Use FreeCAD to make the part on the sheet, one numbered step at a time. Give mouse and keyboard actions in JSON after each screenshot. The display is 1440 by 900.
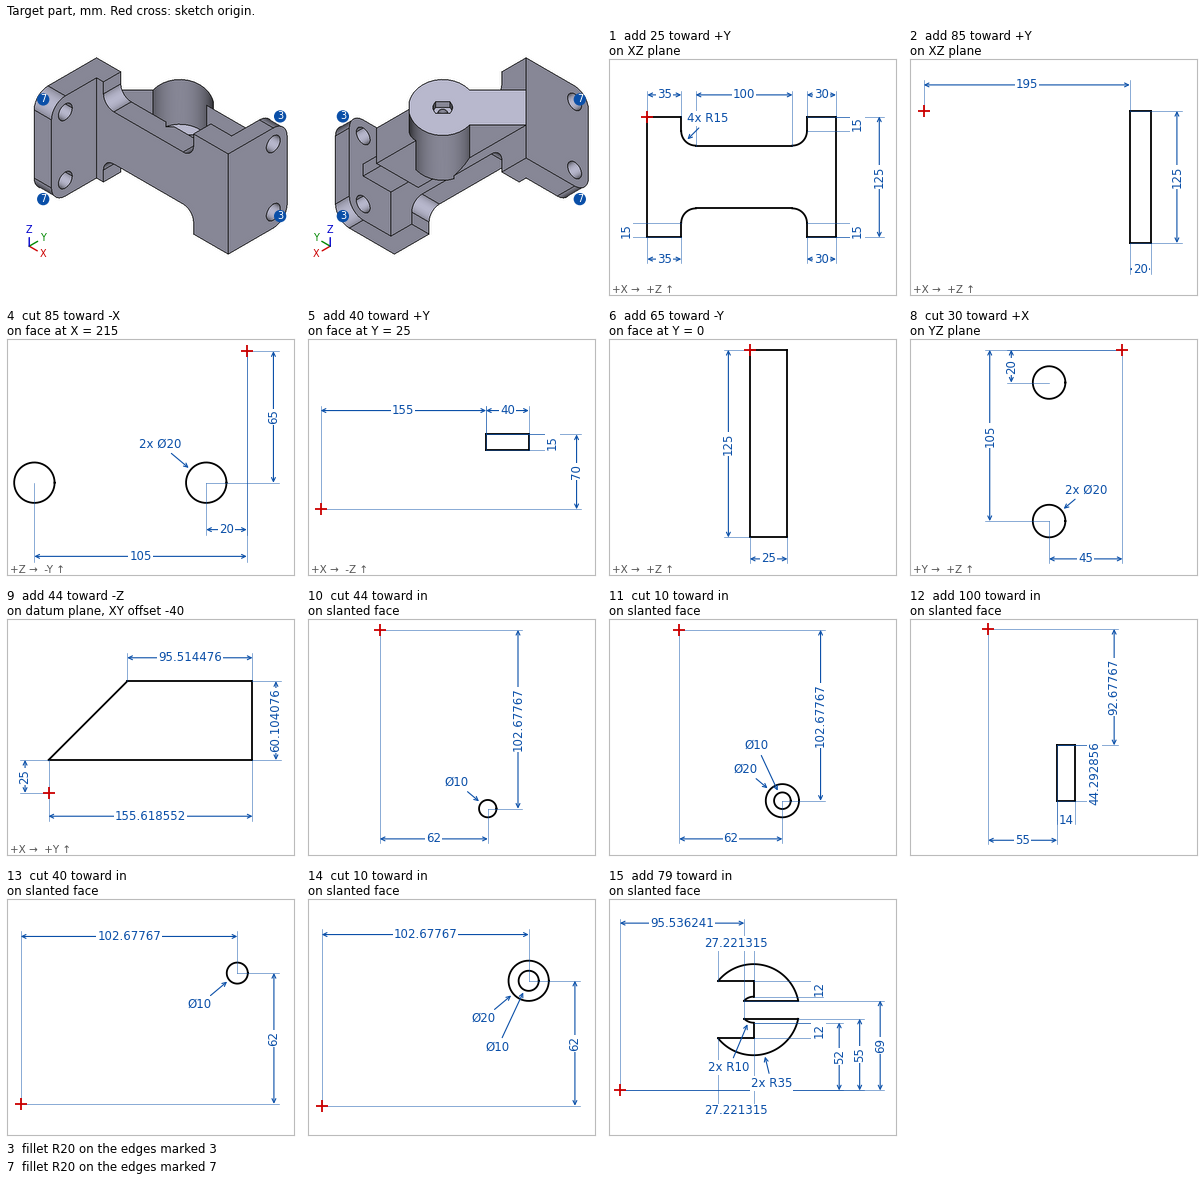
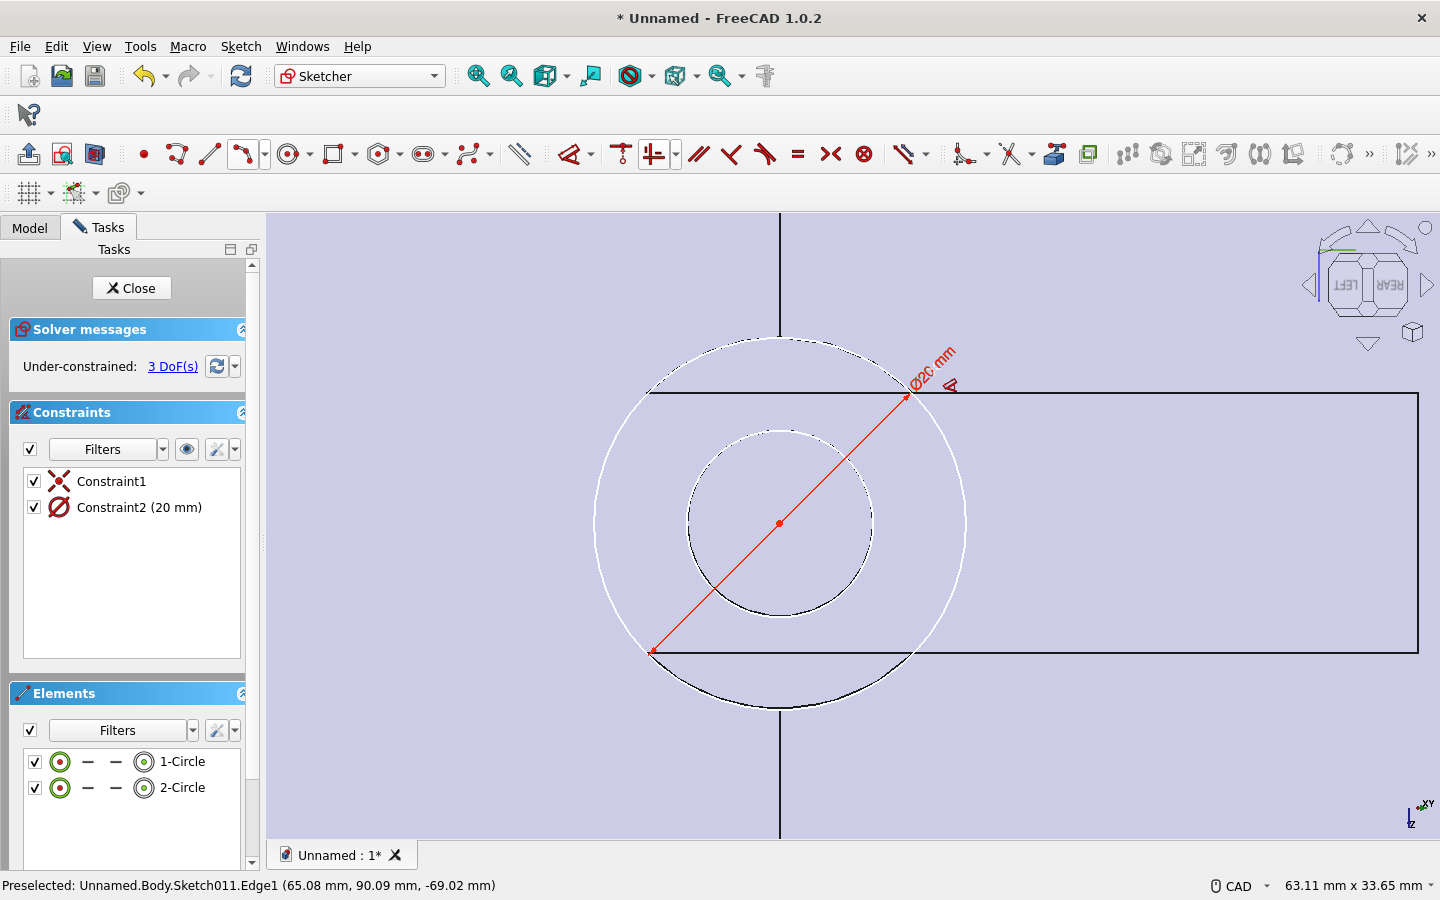
{"action": "left_click", "coordinate": [846, 458]}
{"action": "left_click", "coordinate": [869, 435]}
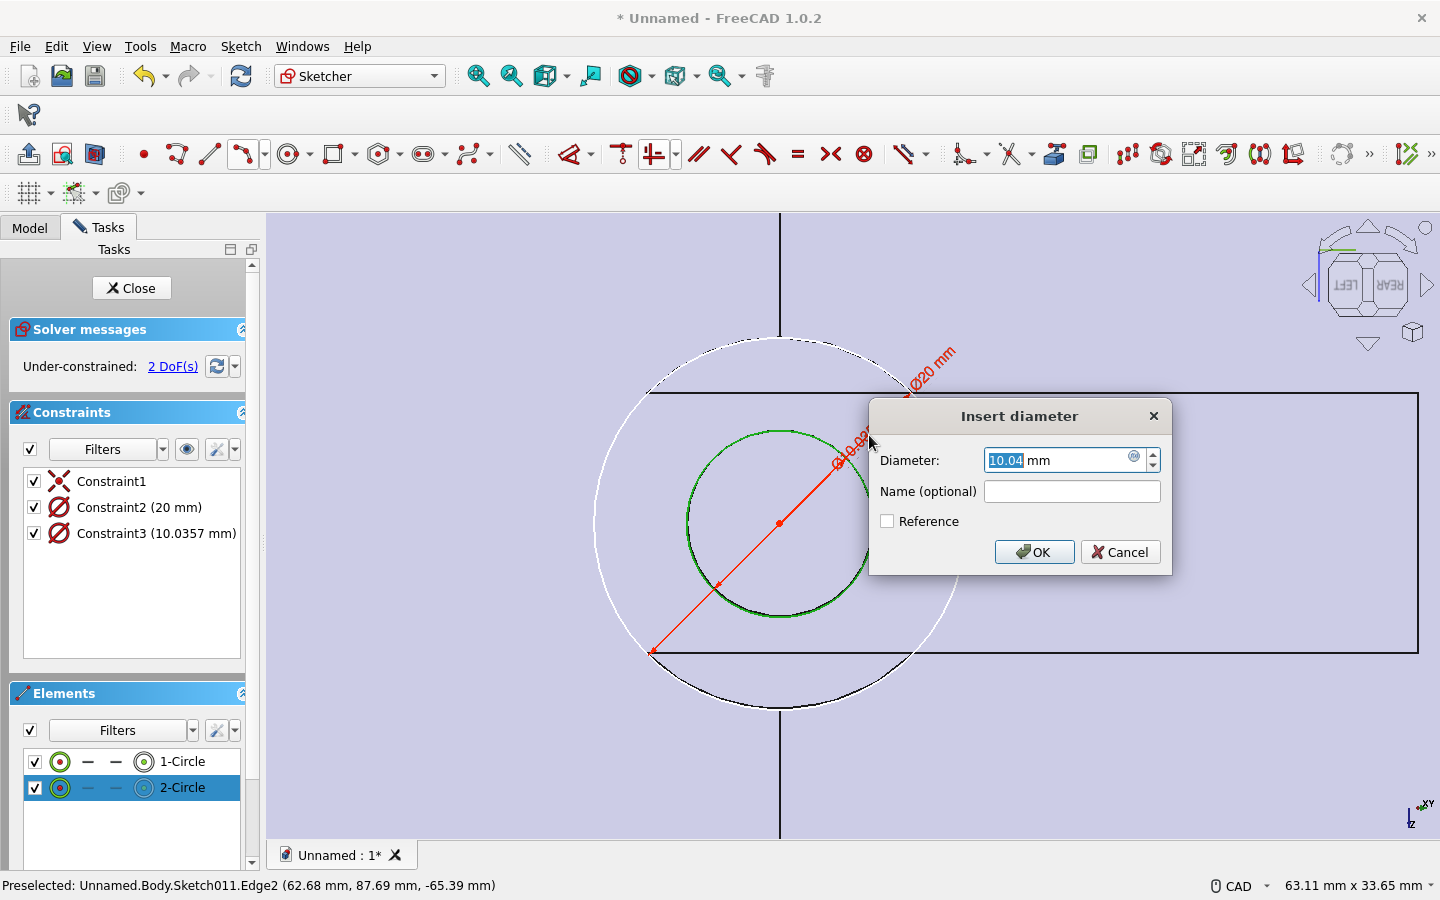
{"action": "type", "text": "10"}
{"action": "key", "text": "Return"}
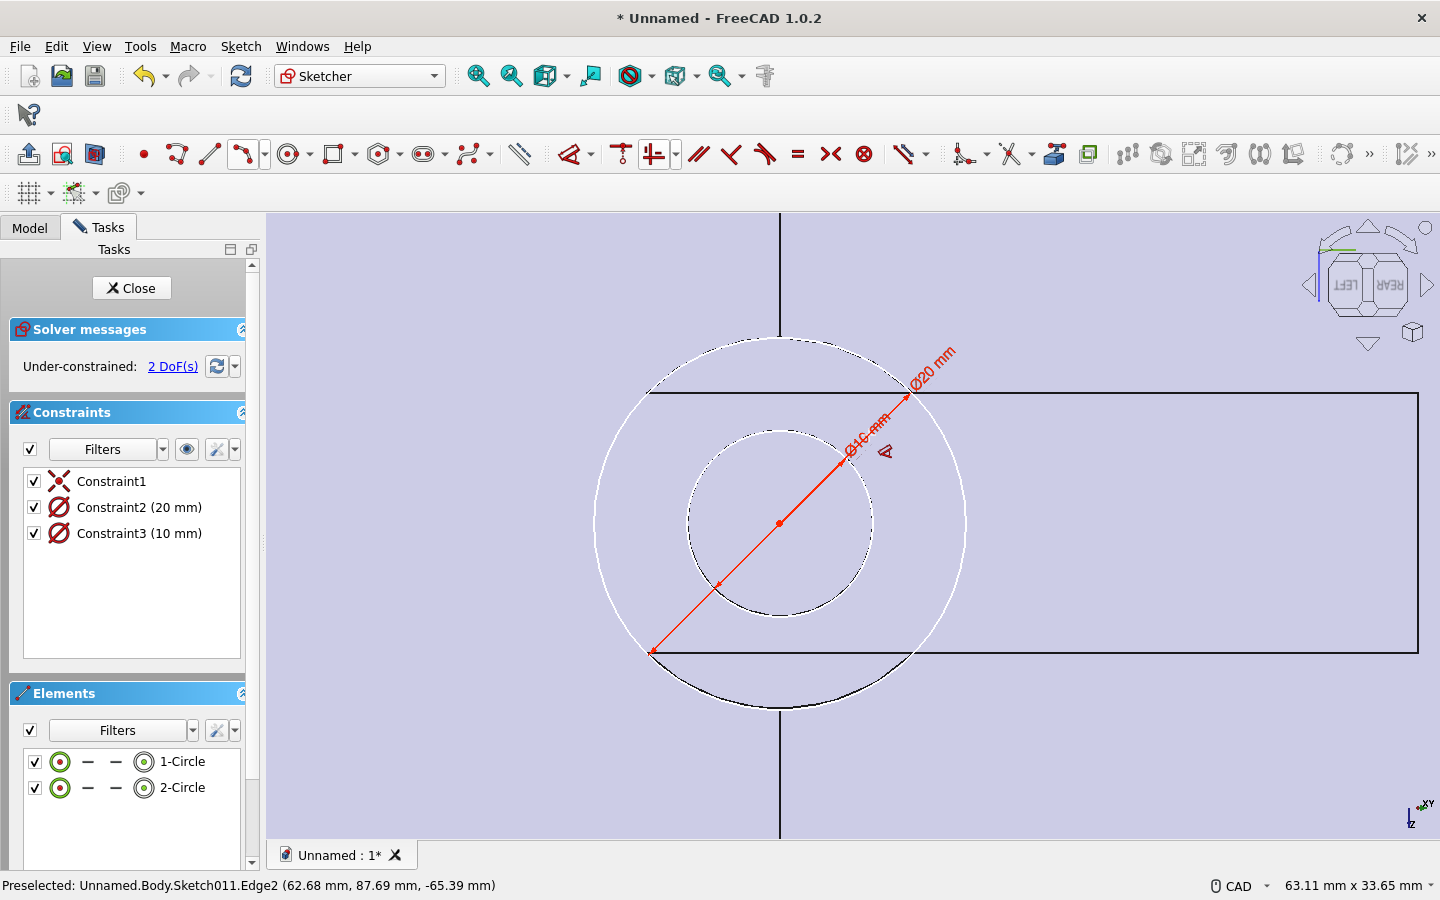
{"action": "left_click", "coordinate": [780, 524]}
{"action": "left_click", "coordinate": [814, 667]}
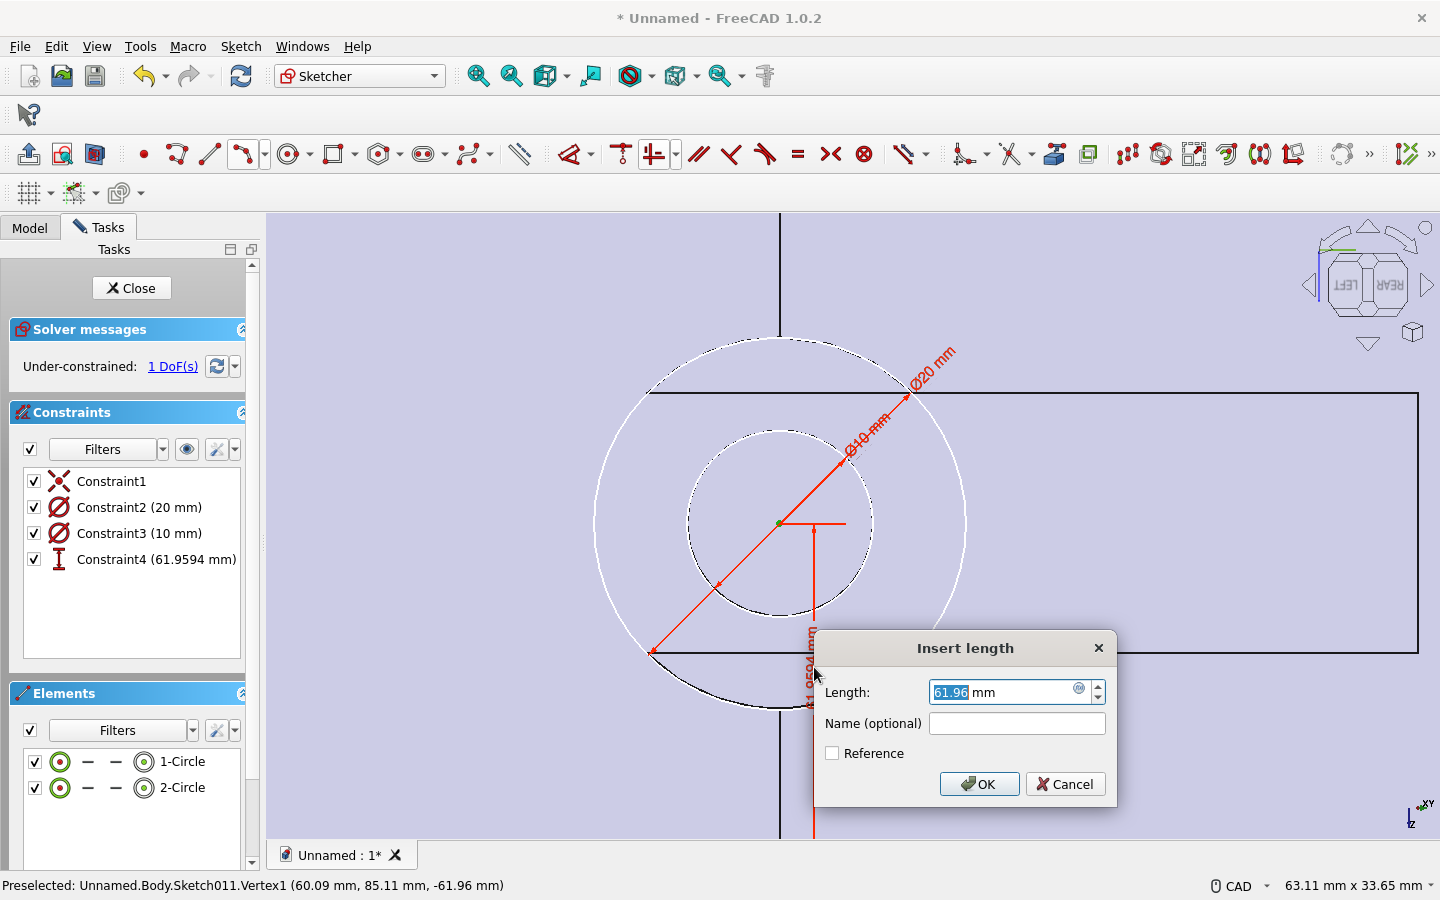
{"action": "type", "text": "62"}
{"action": "key", "text": "Return"}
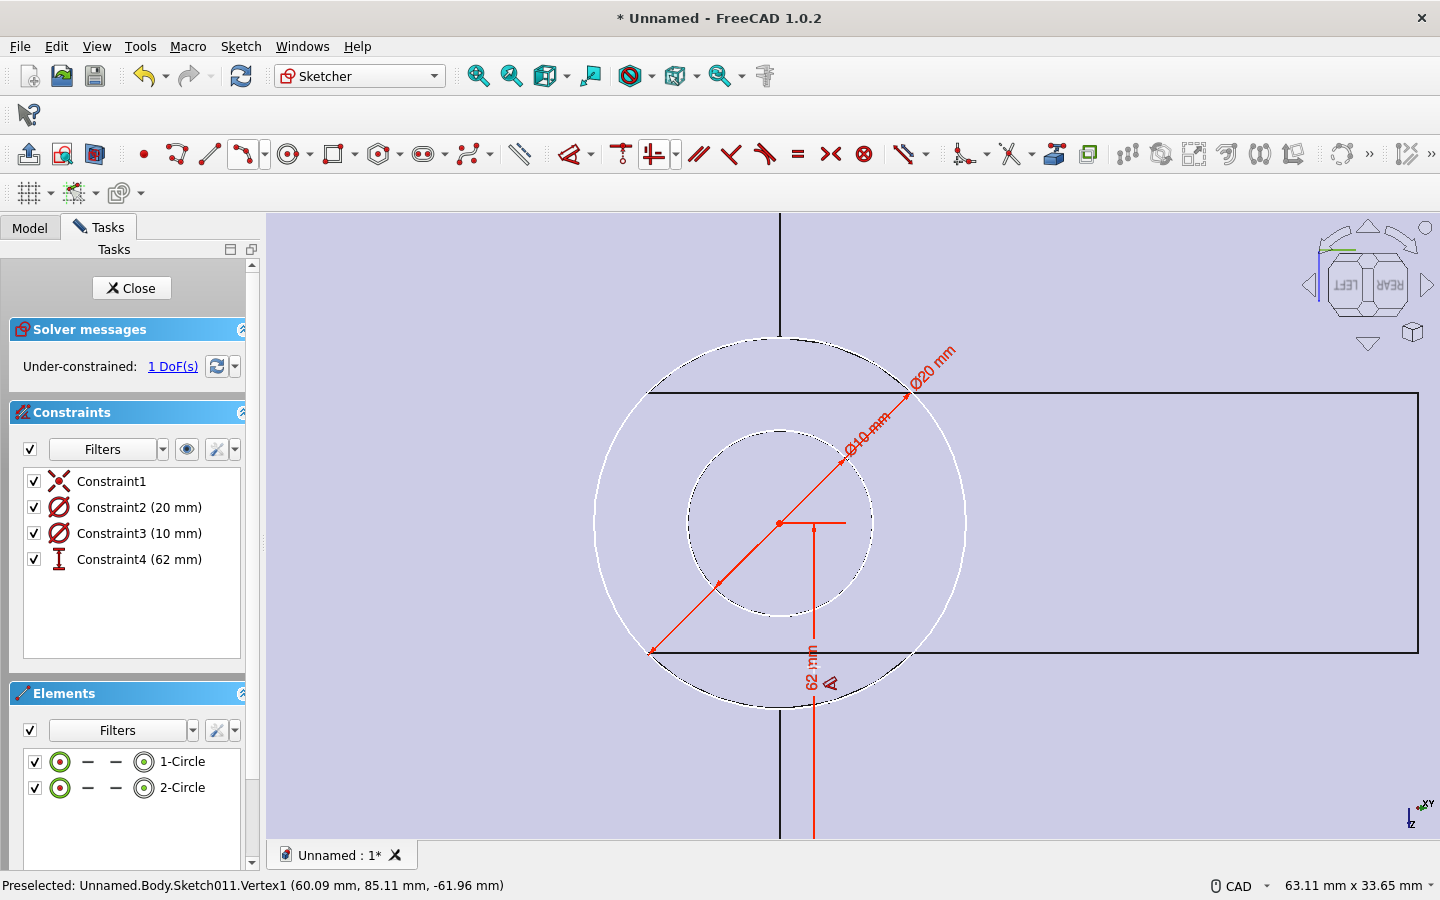
{"action": "left_click", "coordinate": [780, 523]}
{"action": "left_click", "coordinate": [537, 489]}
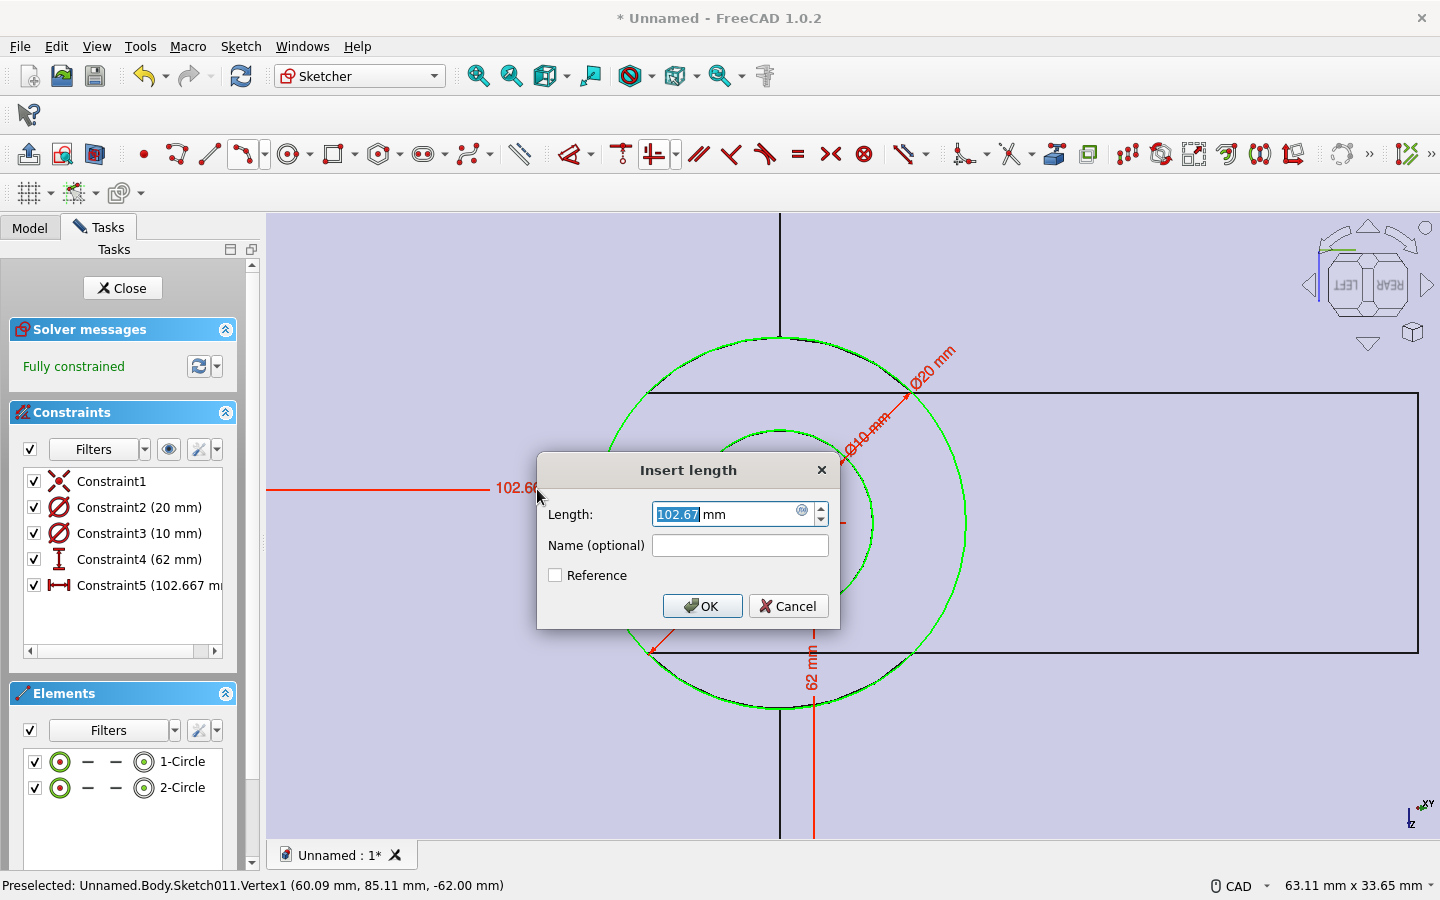
{"action": "type", "text": "102.67767"}
{"action": "key", "text": "Return"}
{"action": "key", "text": "Escape"}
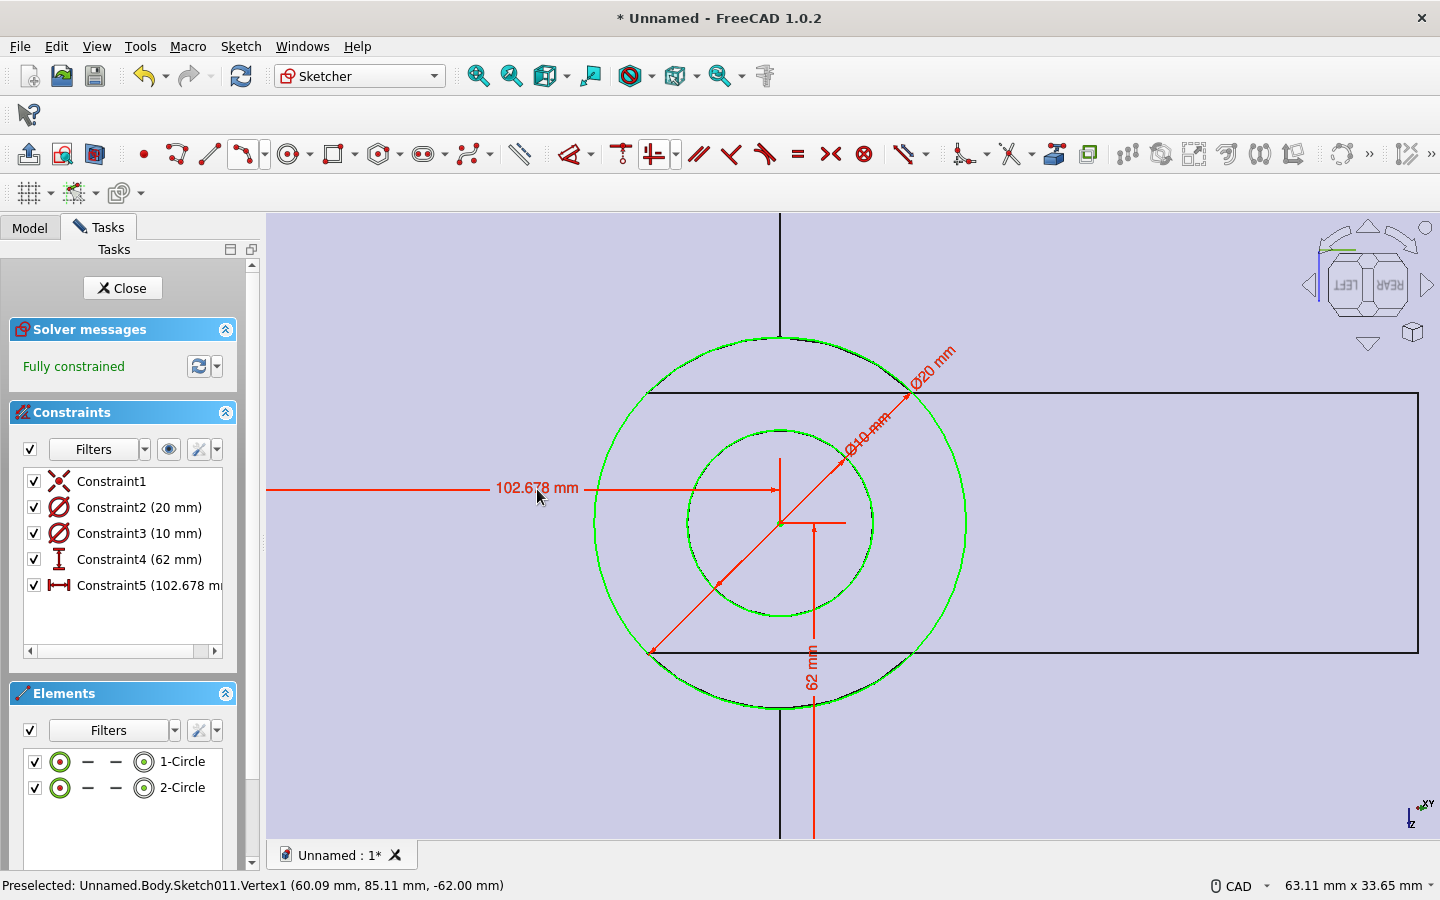
{"action": "left_click", "coordinate": [123, 288]}